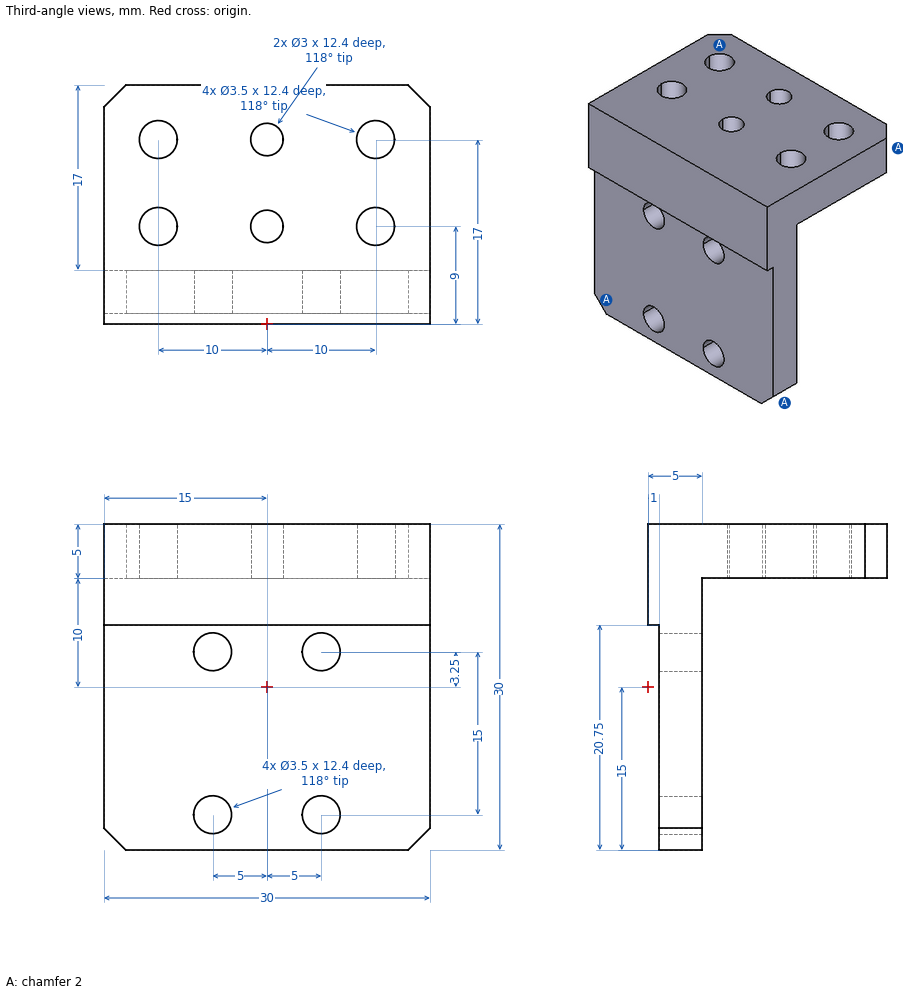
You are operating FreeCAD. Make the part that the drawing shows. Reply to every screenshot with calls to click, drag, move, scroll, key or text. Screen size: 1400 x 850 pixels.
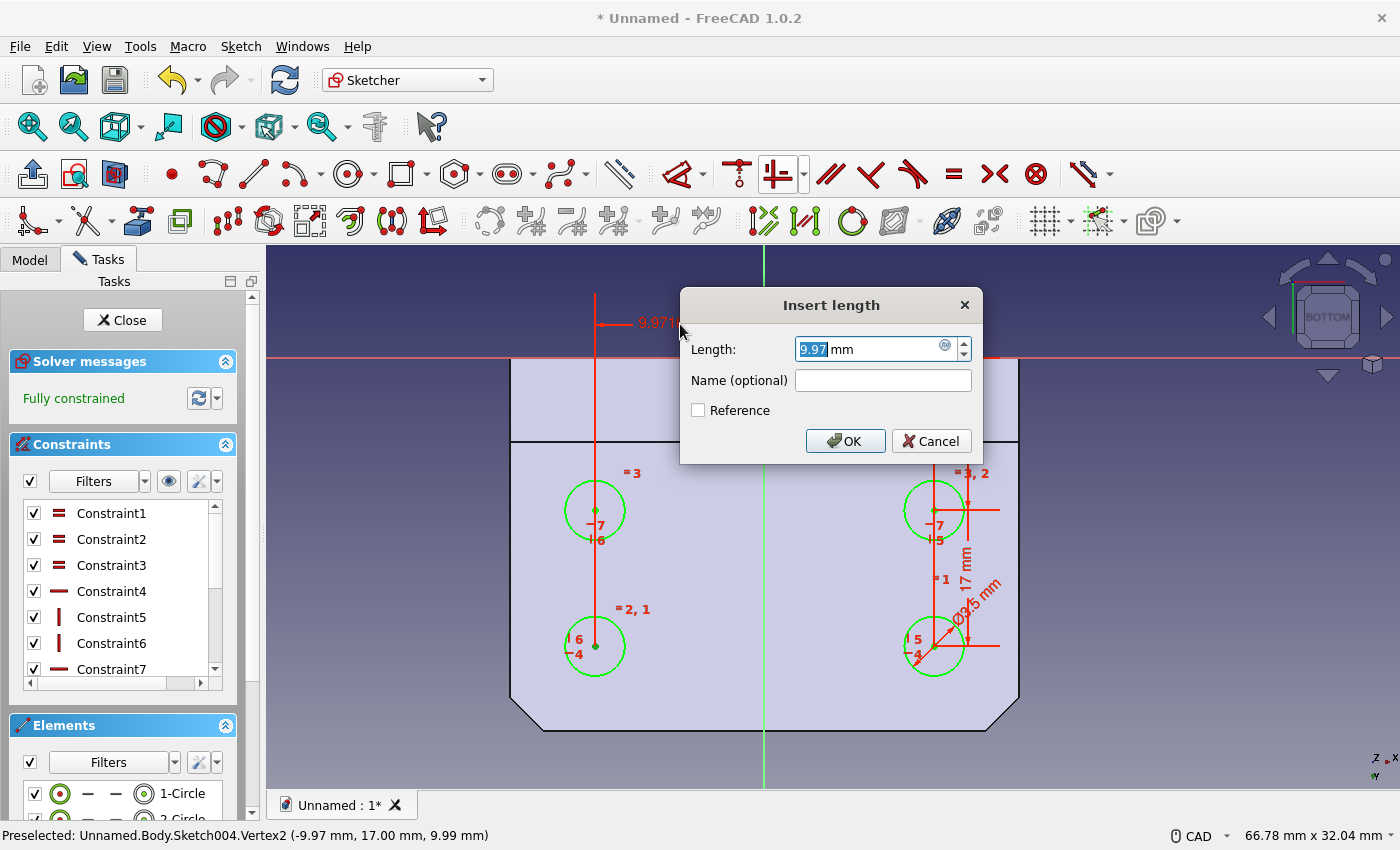
text(10)
key(Return)
key(Escape)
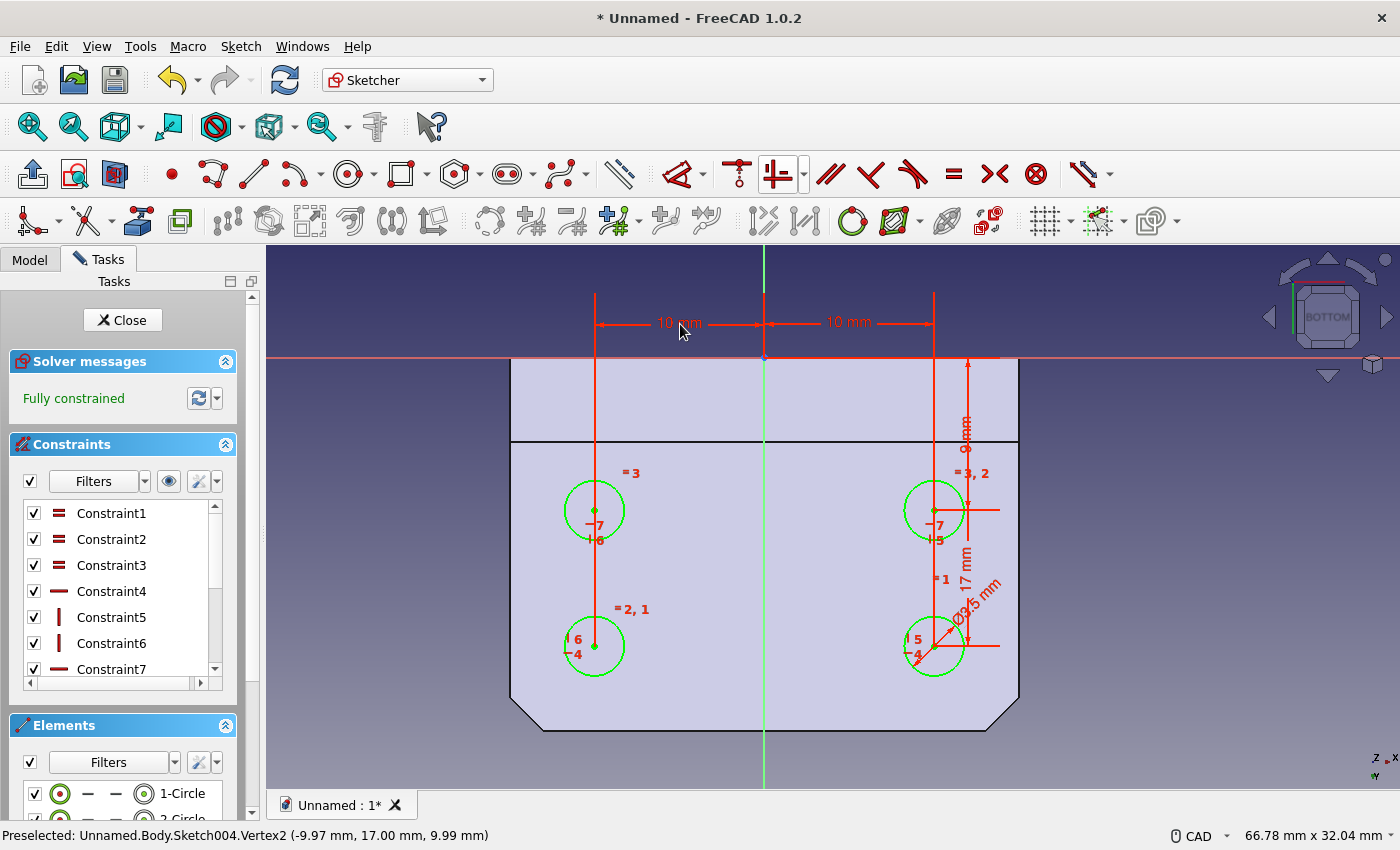
click(123, 320)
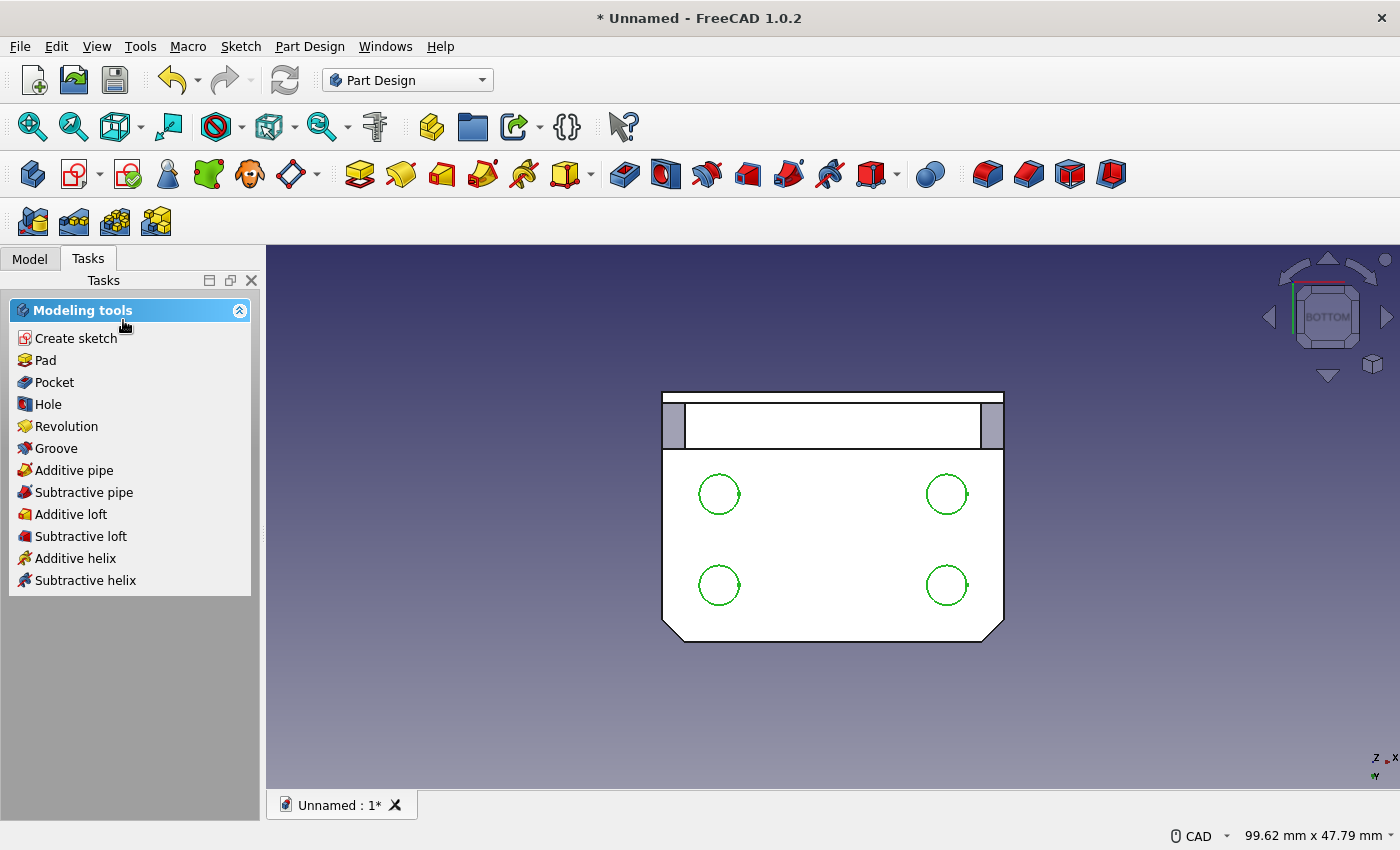
click(666, 174)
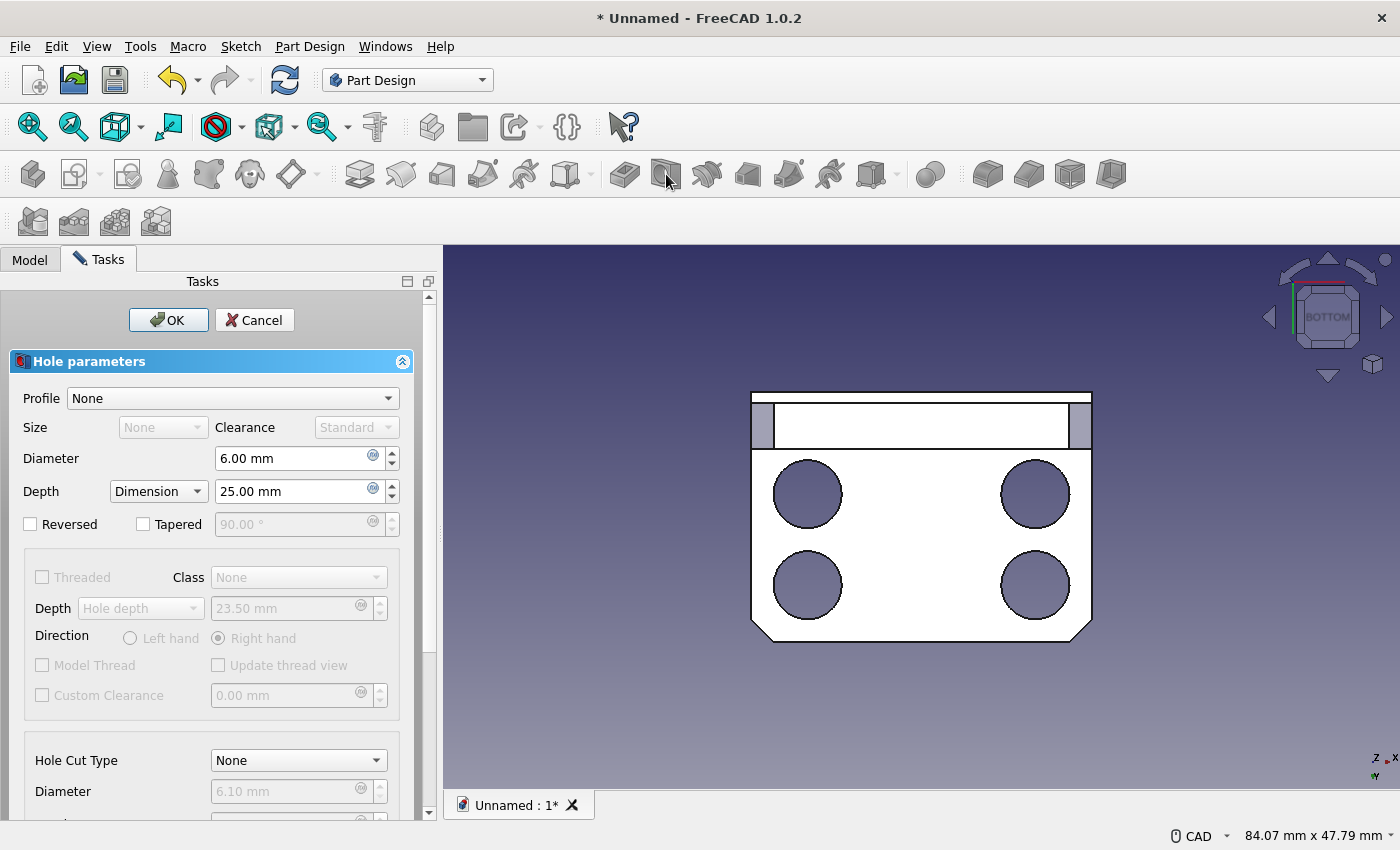
triple_click(300, 458)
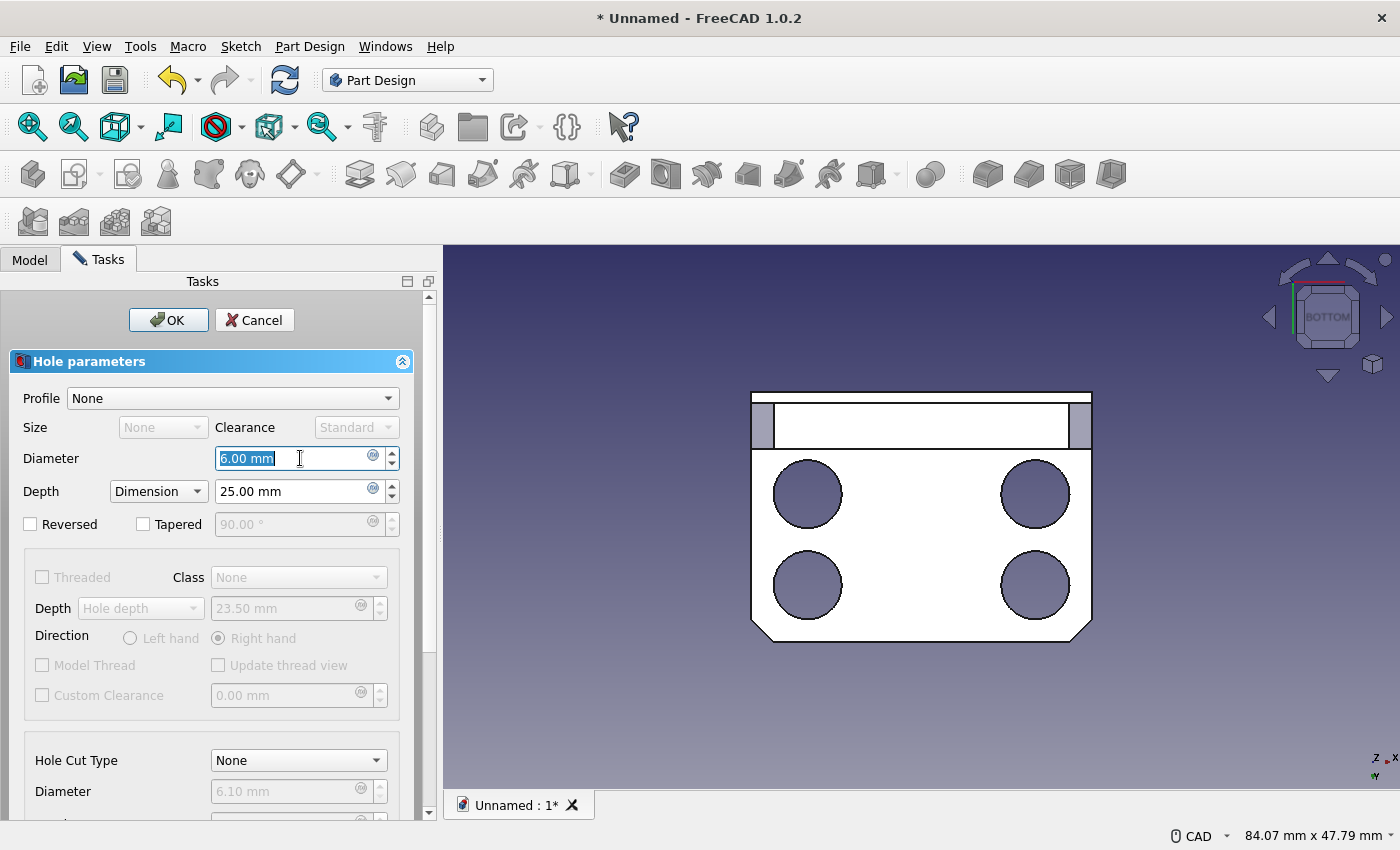
text(3.5)
key(Tab)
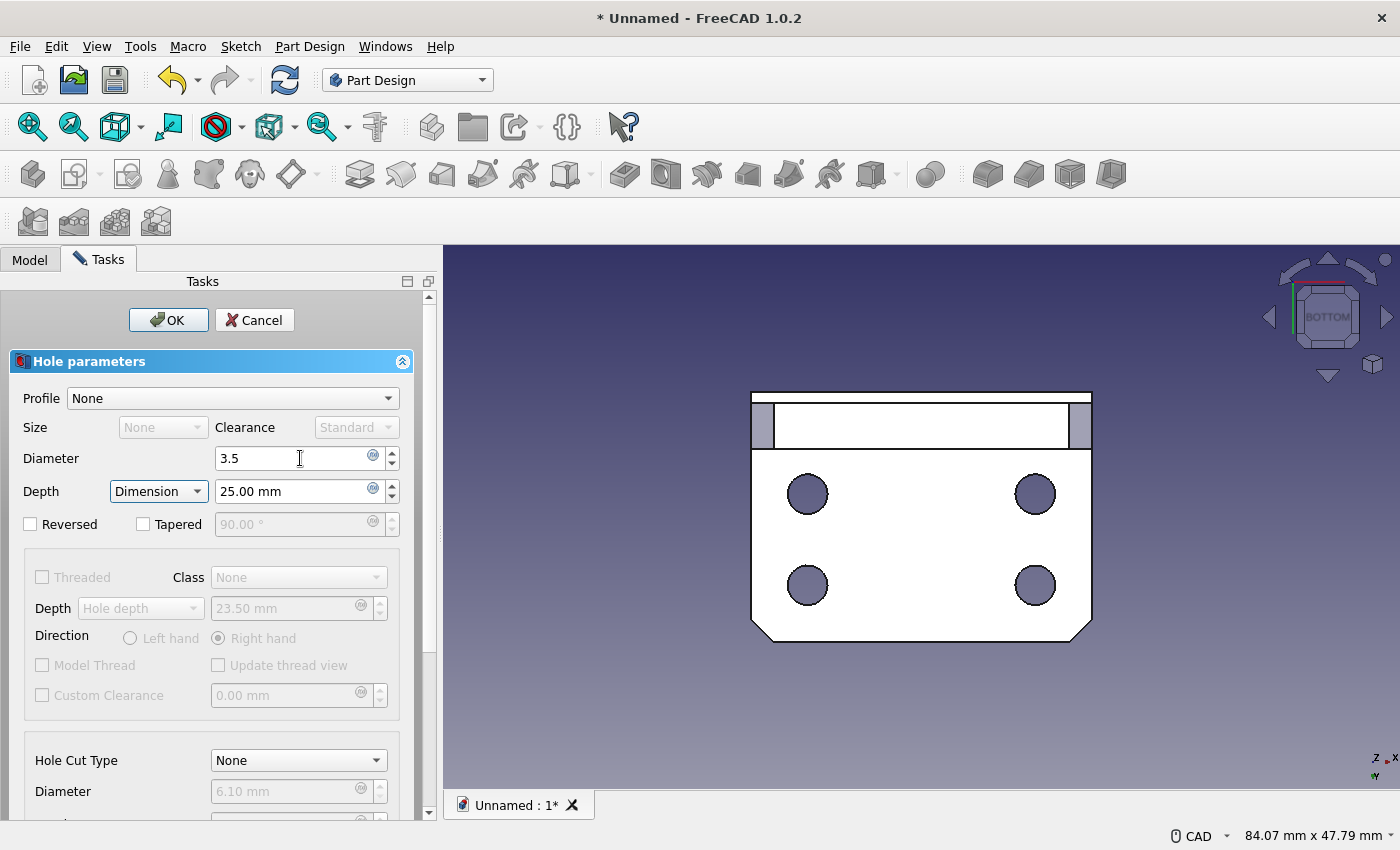
triple_click(300, 492)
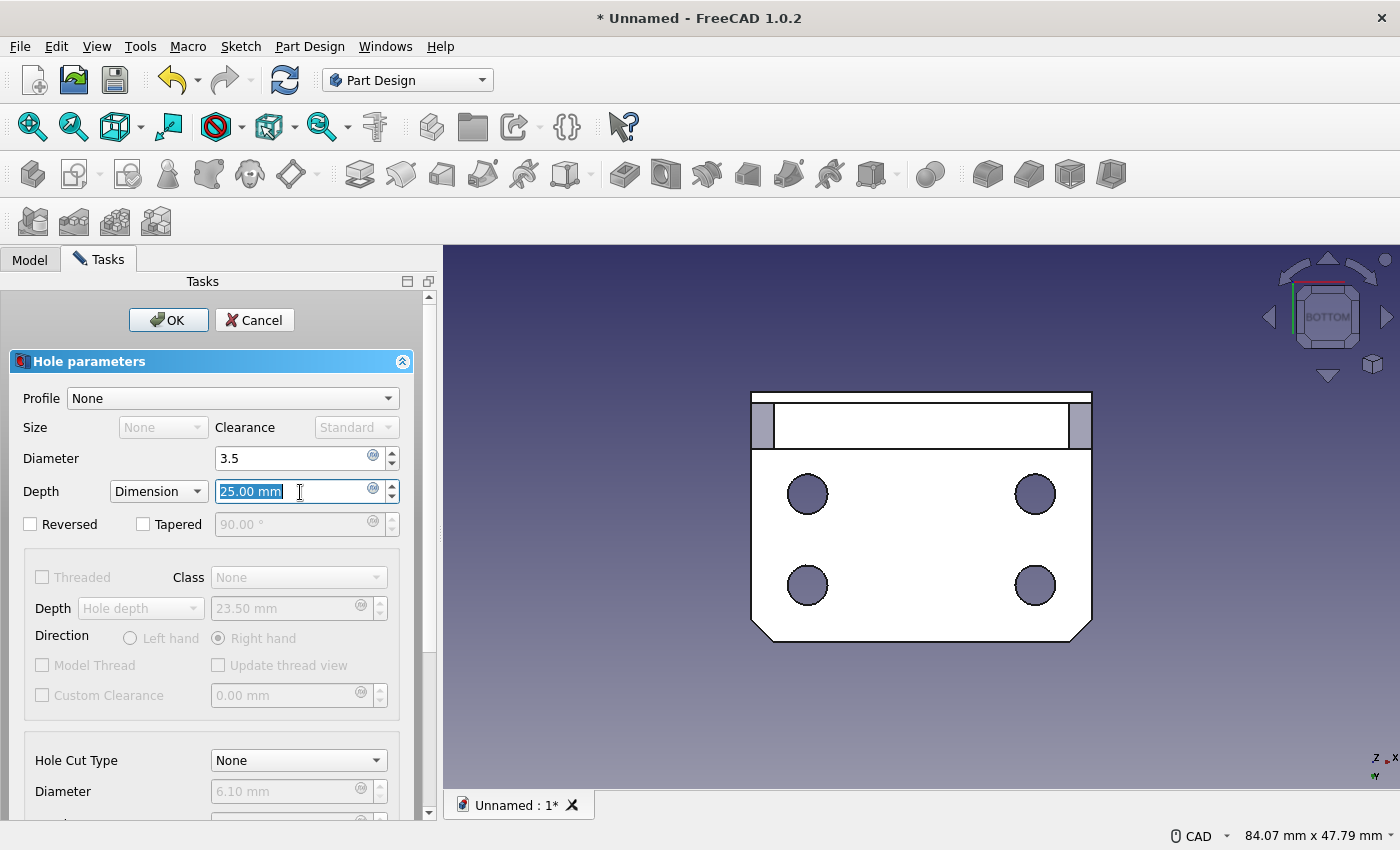
text(12.4)
key(Tab)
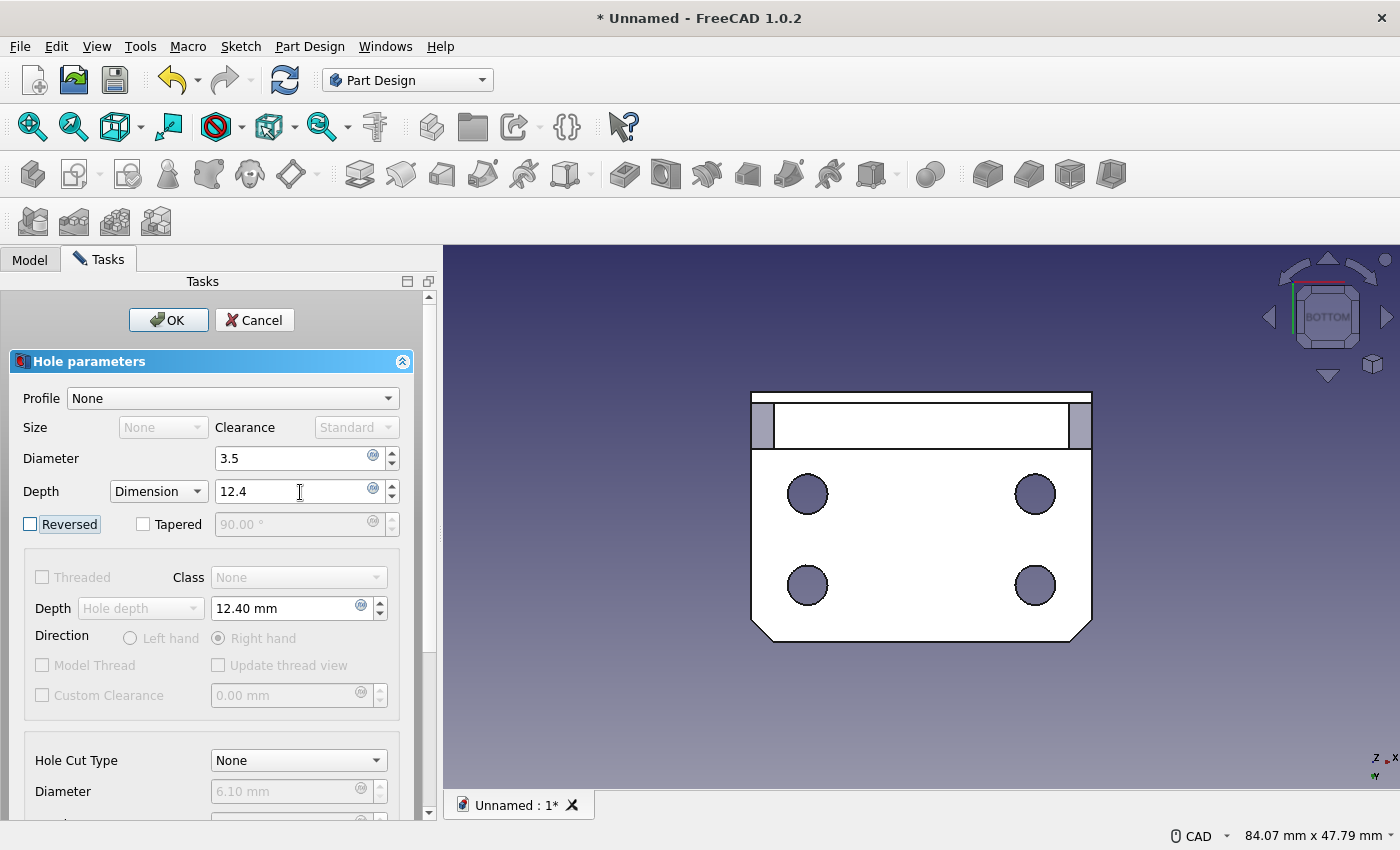
click(169, 320)